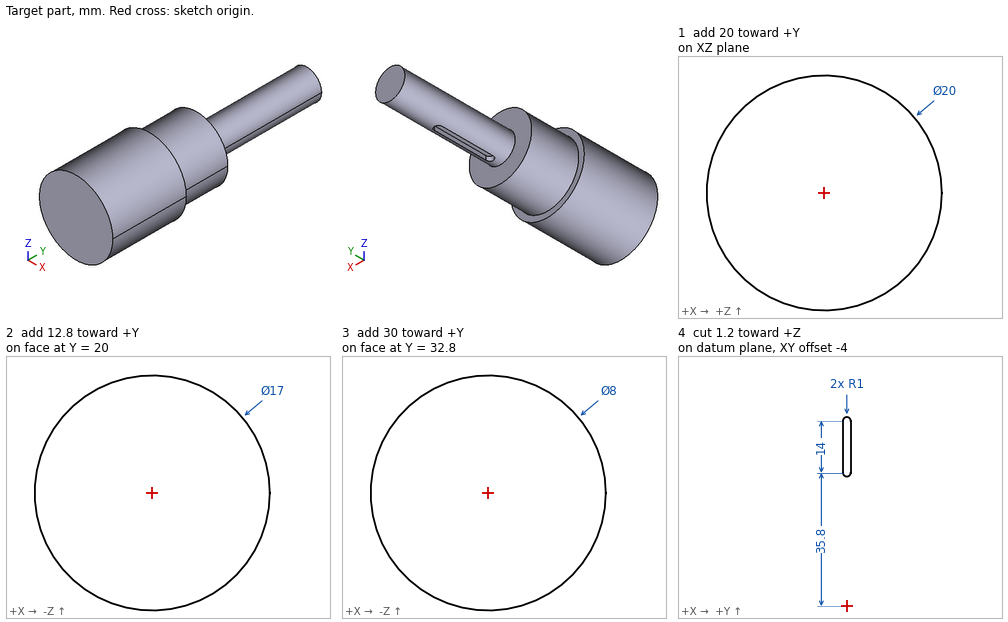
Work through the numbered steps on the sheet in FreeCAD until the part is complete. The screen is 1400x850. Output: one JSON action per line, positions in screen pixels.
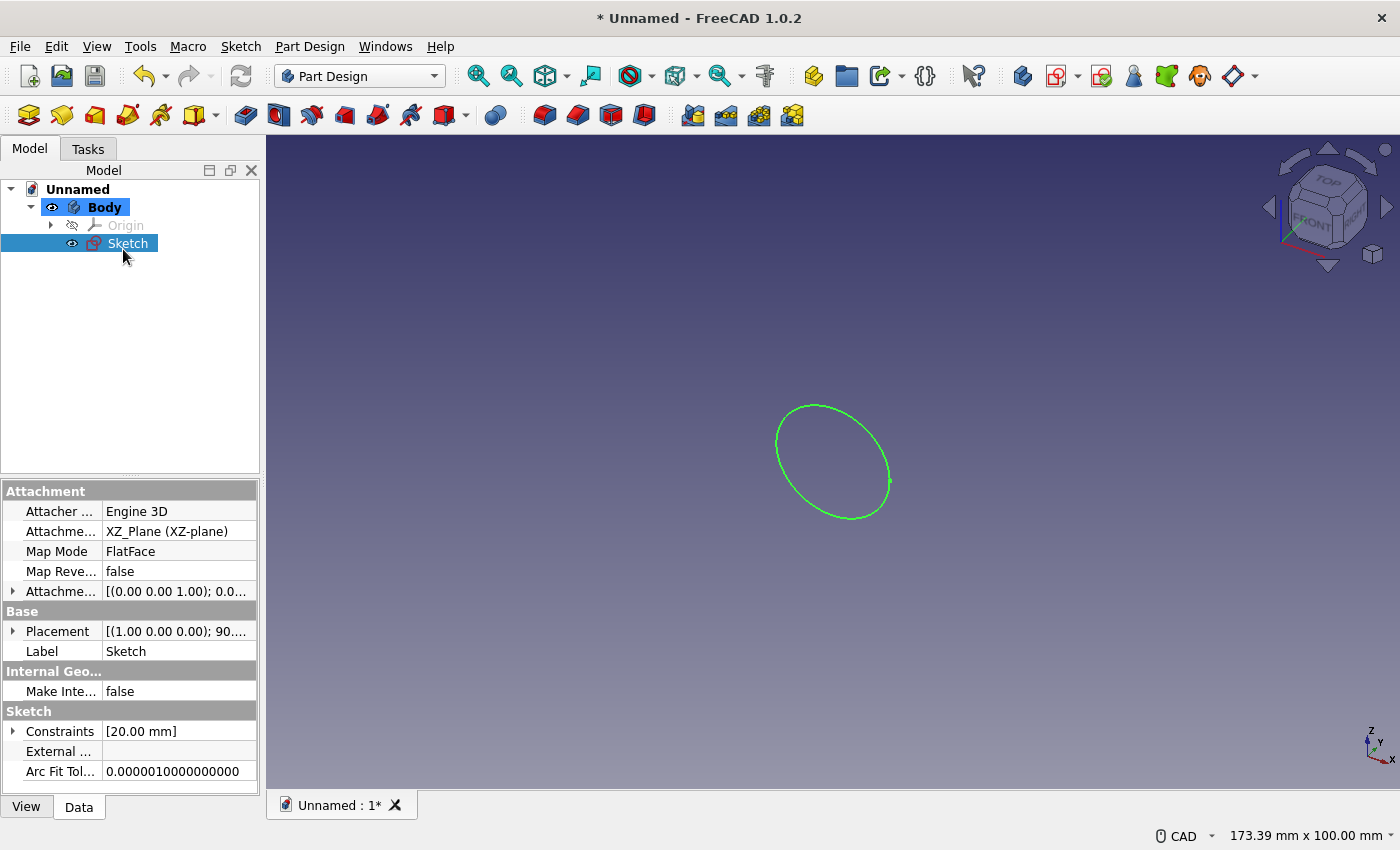
{"action": "left_click", "coordinate": [29, 116]}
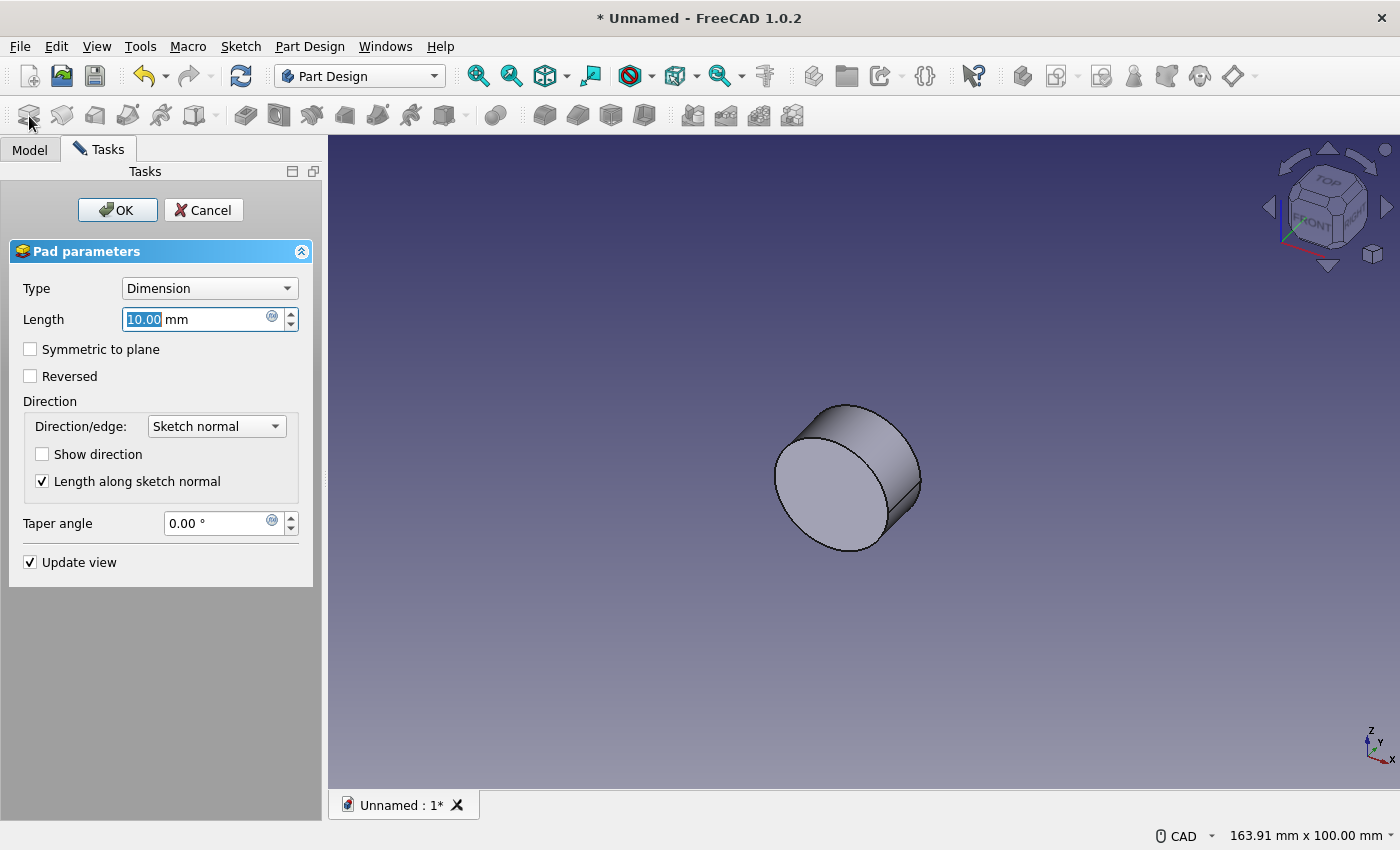
{"action": "type", "text": "20"}
{"action": "key", "text": "Tab"}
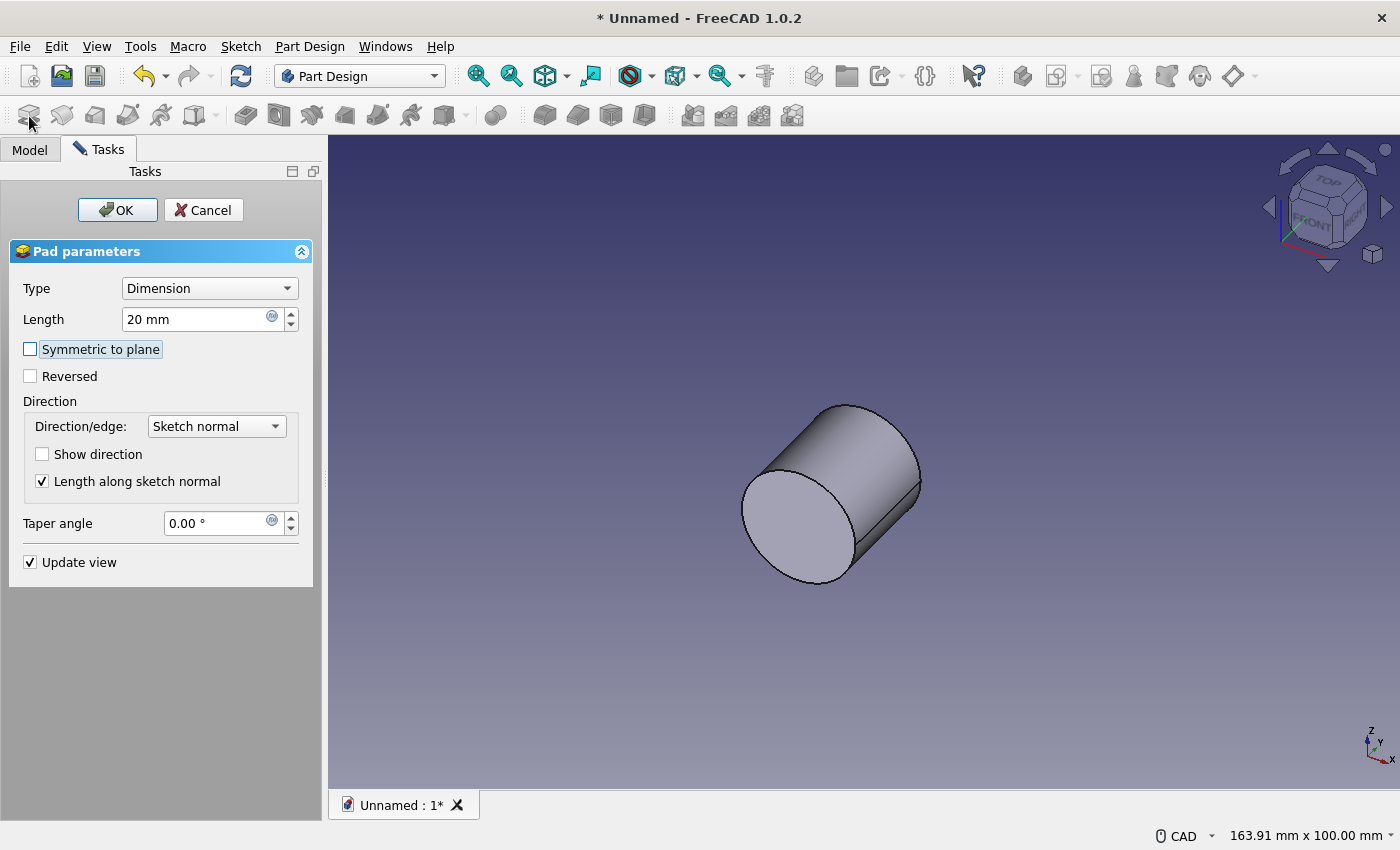
{"action": "left_click", "coordinate": [31, 376]}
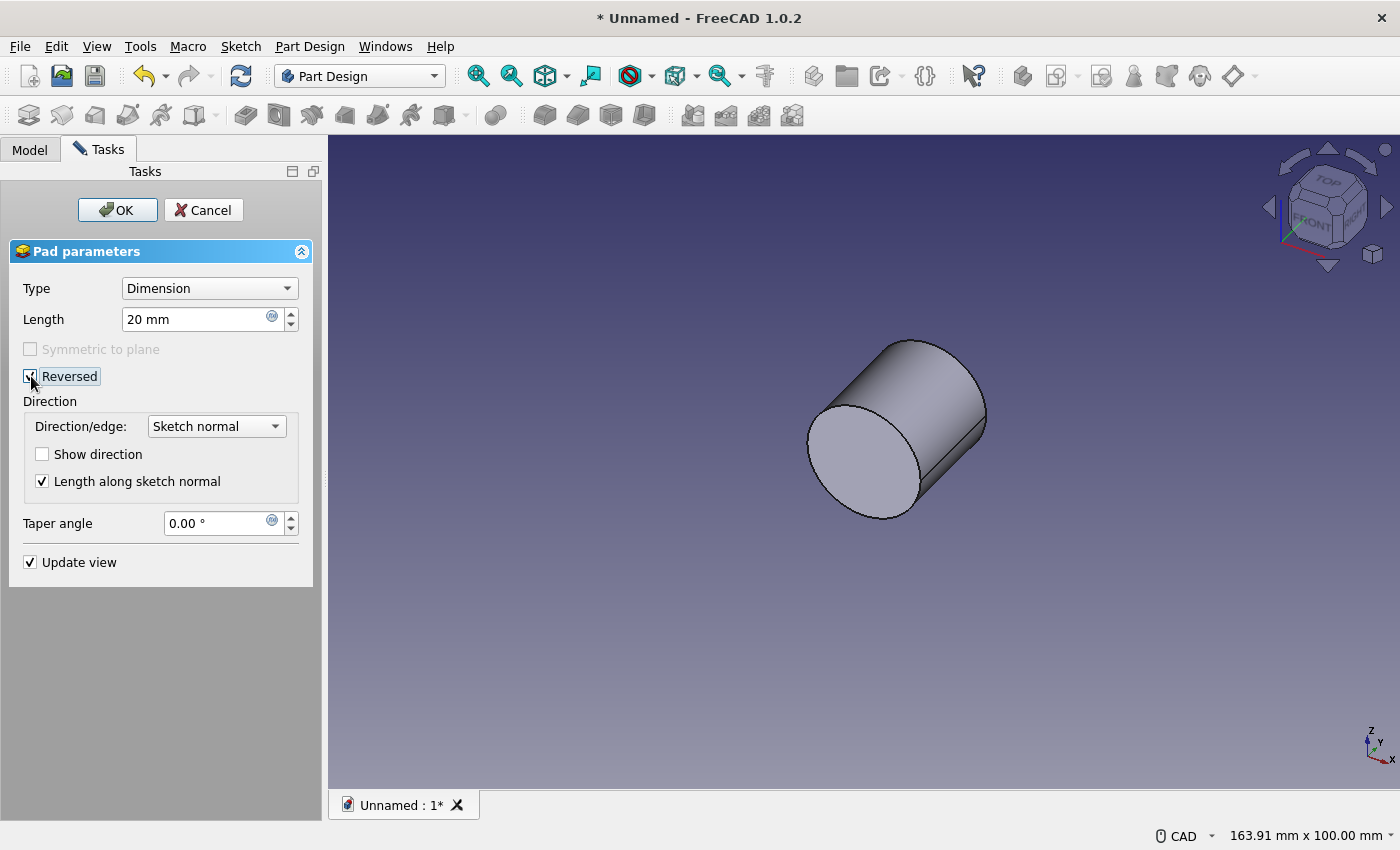
{"action": "left_click", "coordinate": [118, 210]}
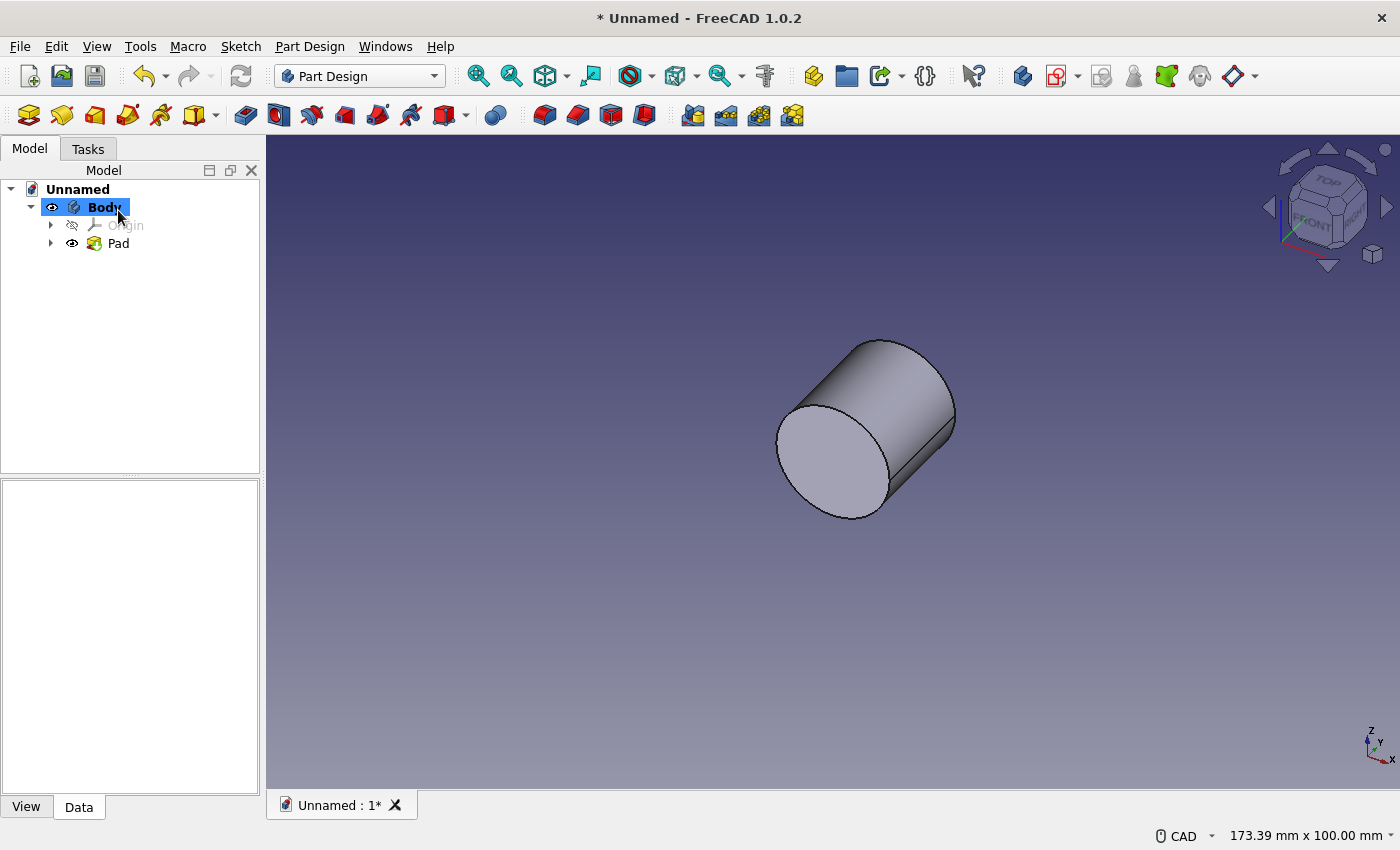
{"action": "left_click", "coordinate": [479, 76]}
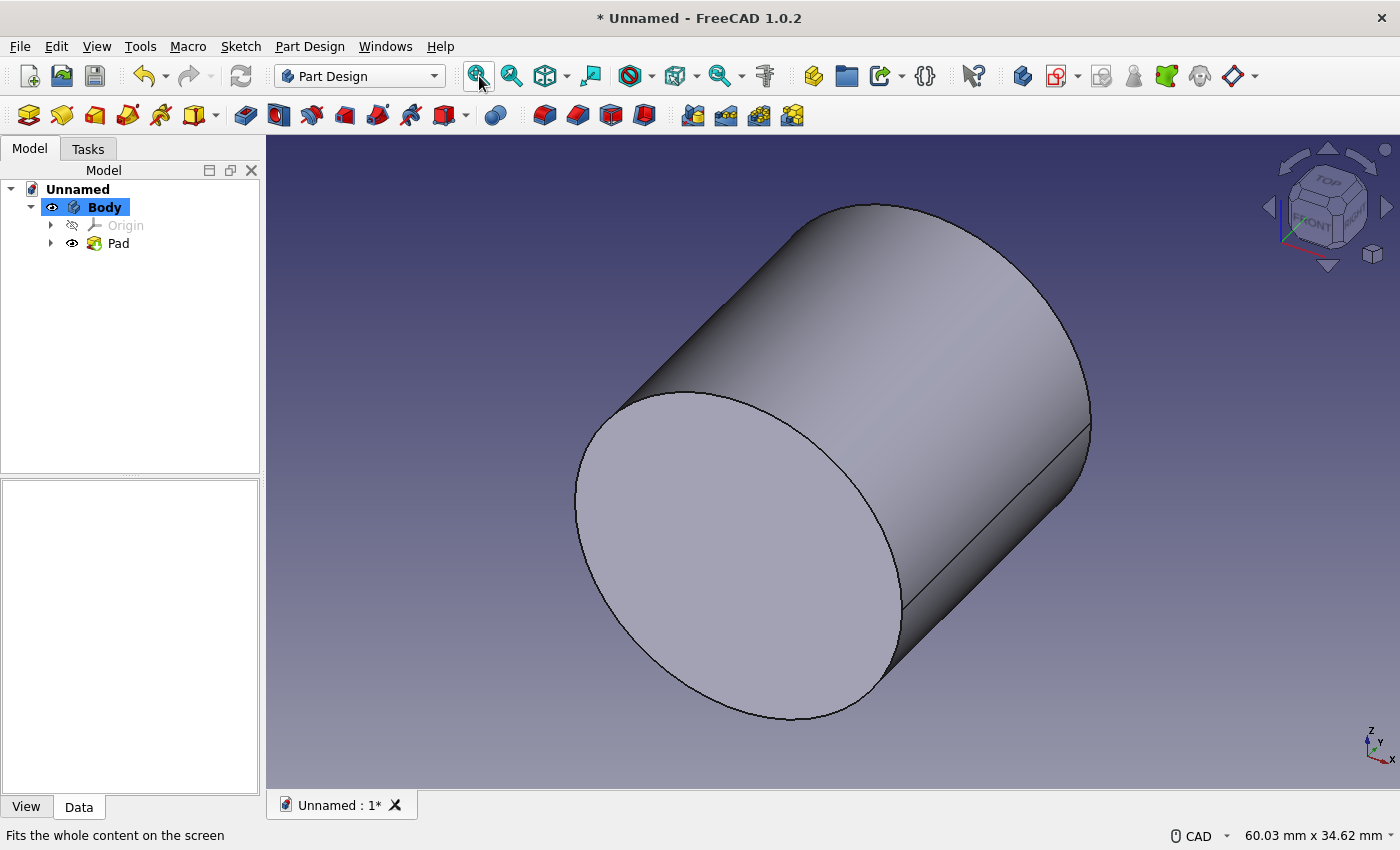
{"action": "key", "text": "4"}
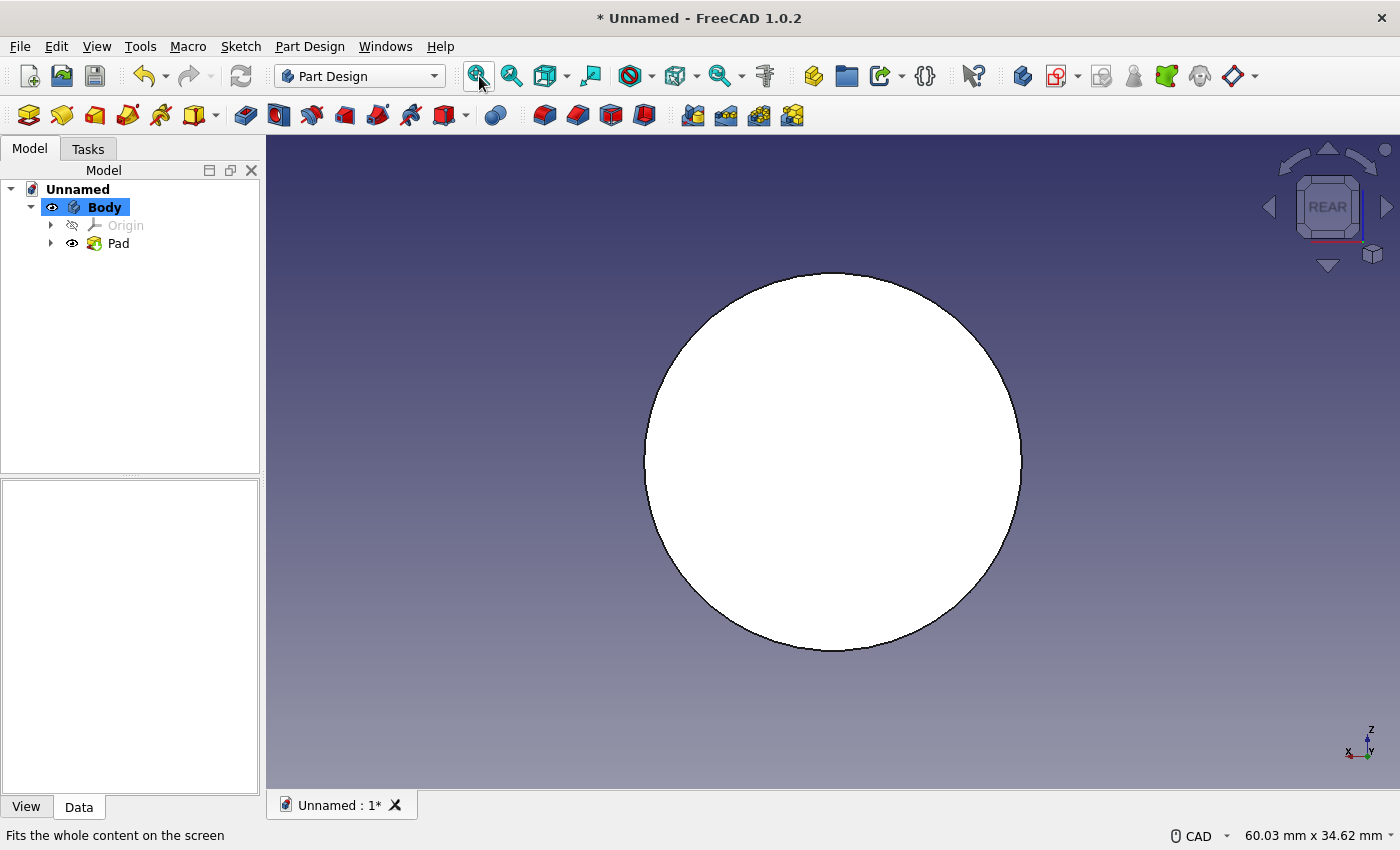
{"action": "left_click", "coordinate": [833, 461]}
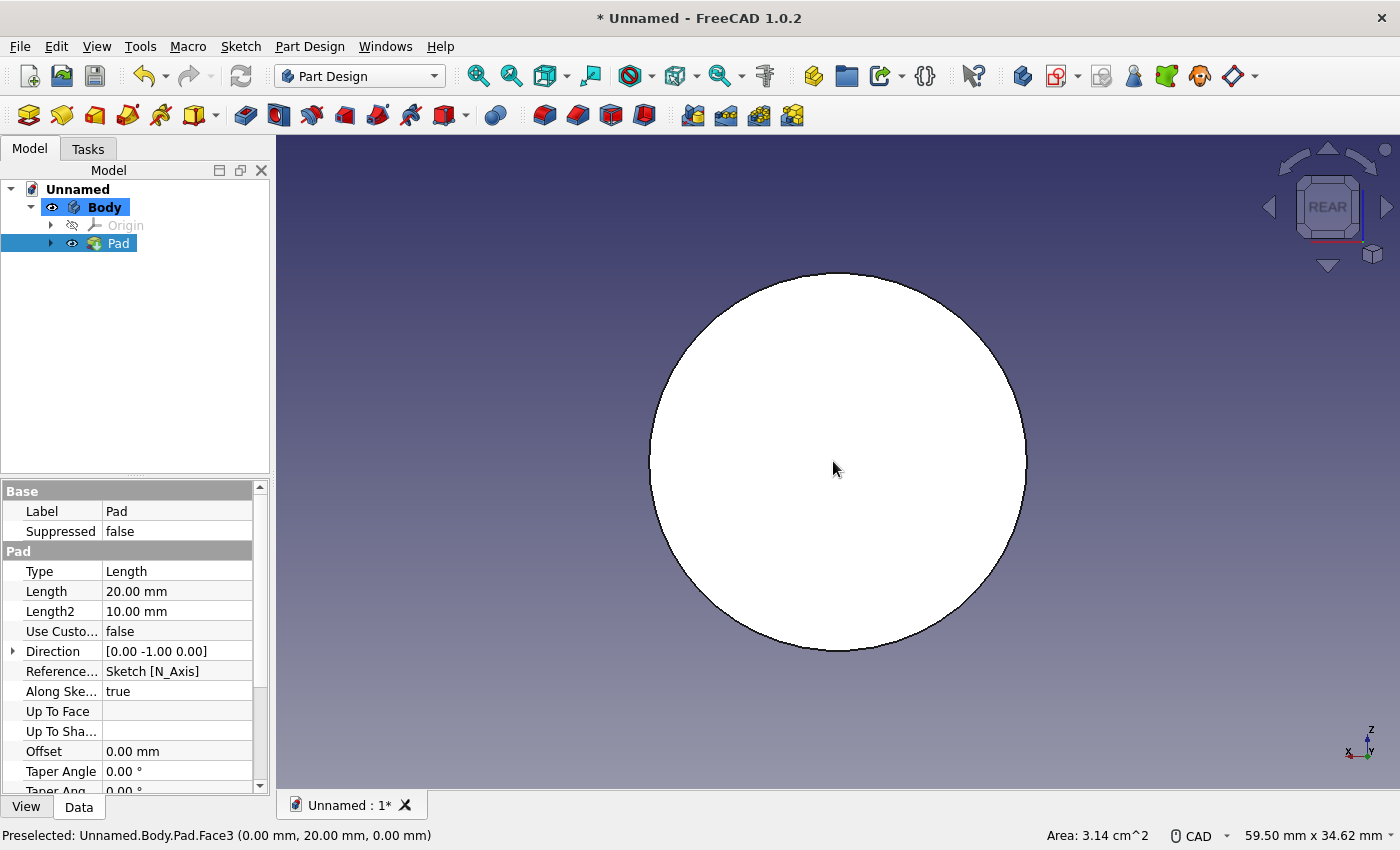
{"action": "left_click", "coordinate": [1056, 76]}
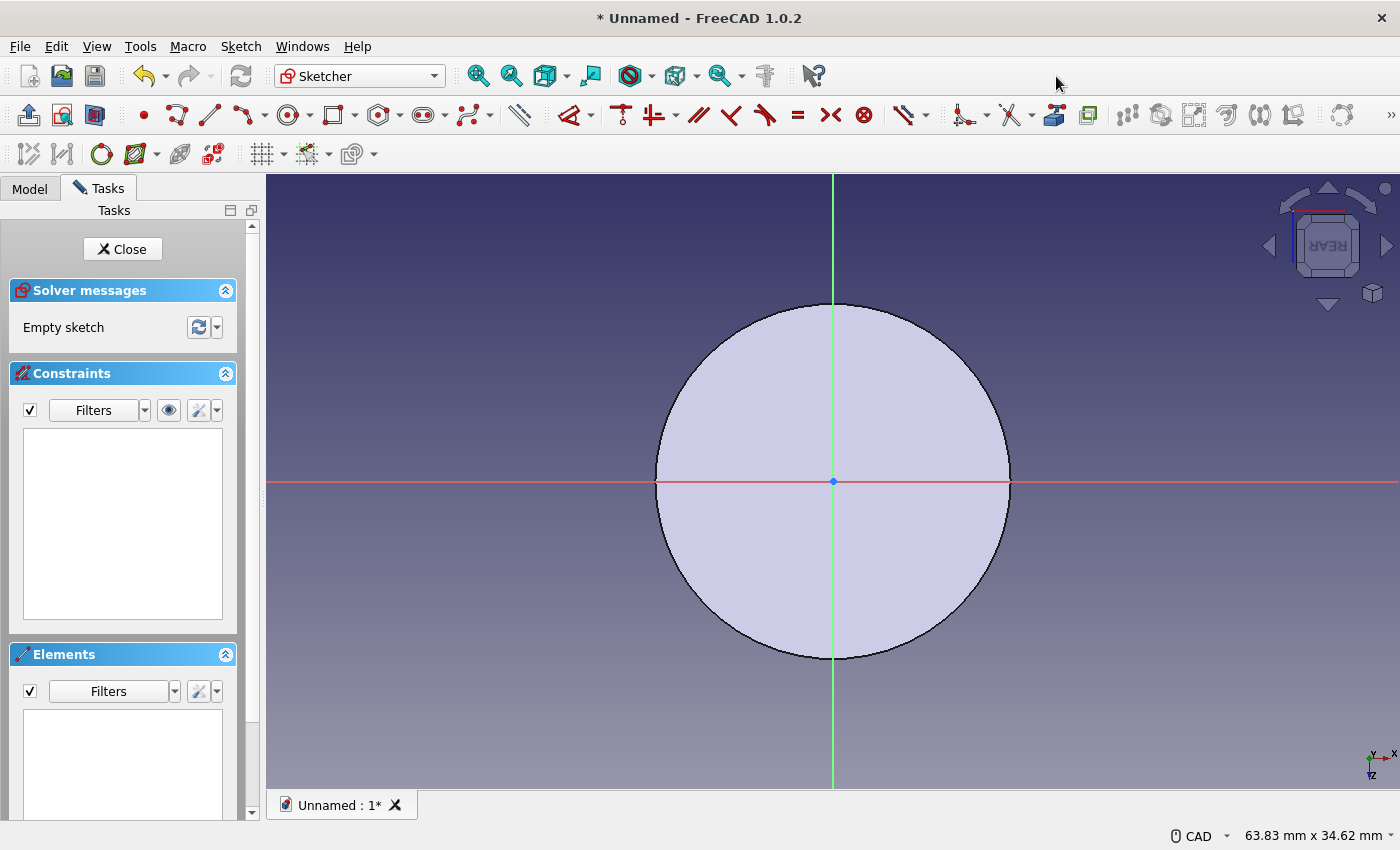
{"action": "left_click", "coordinate": [288, 116]}